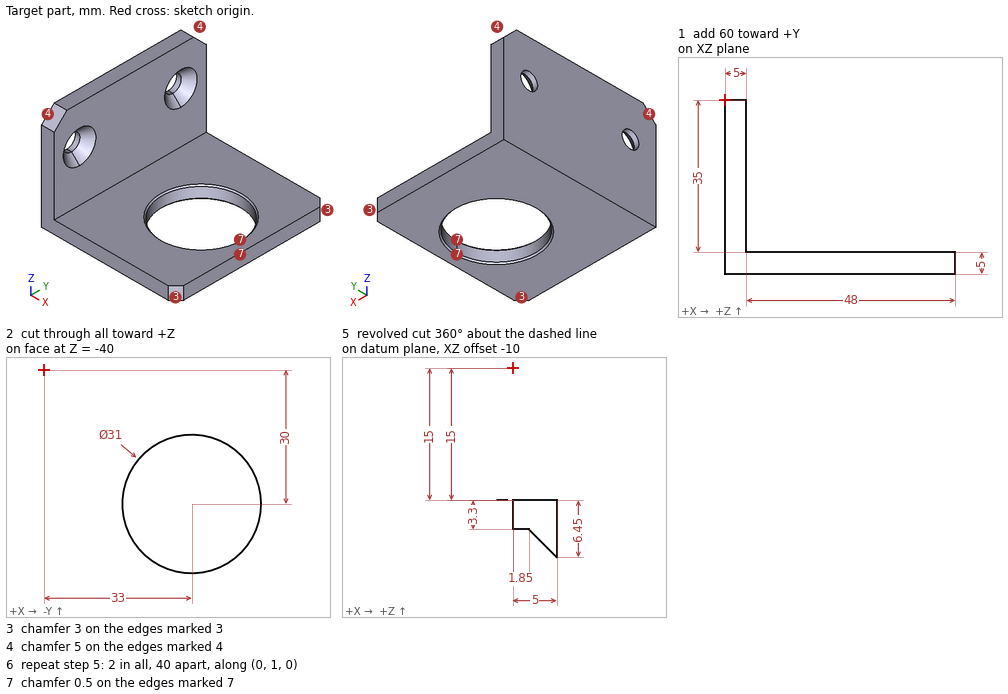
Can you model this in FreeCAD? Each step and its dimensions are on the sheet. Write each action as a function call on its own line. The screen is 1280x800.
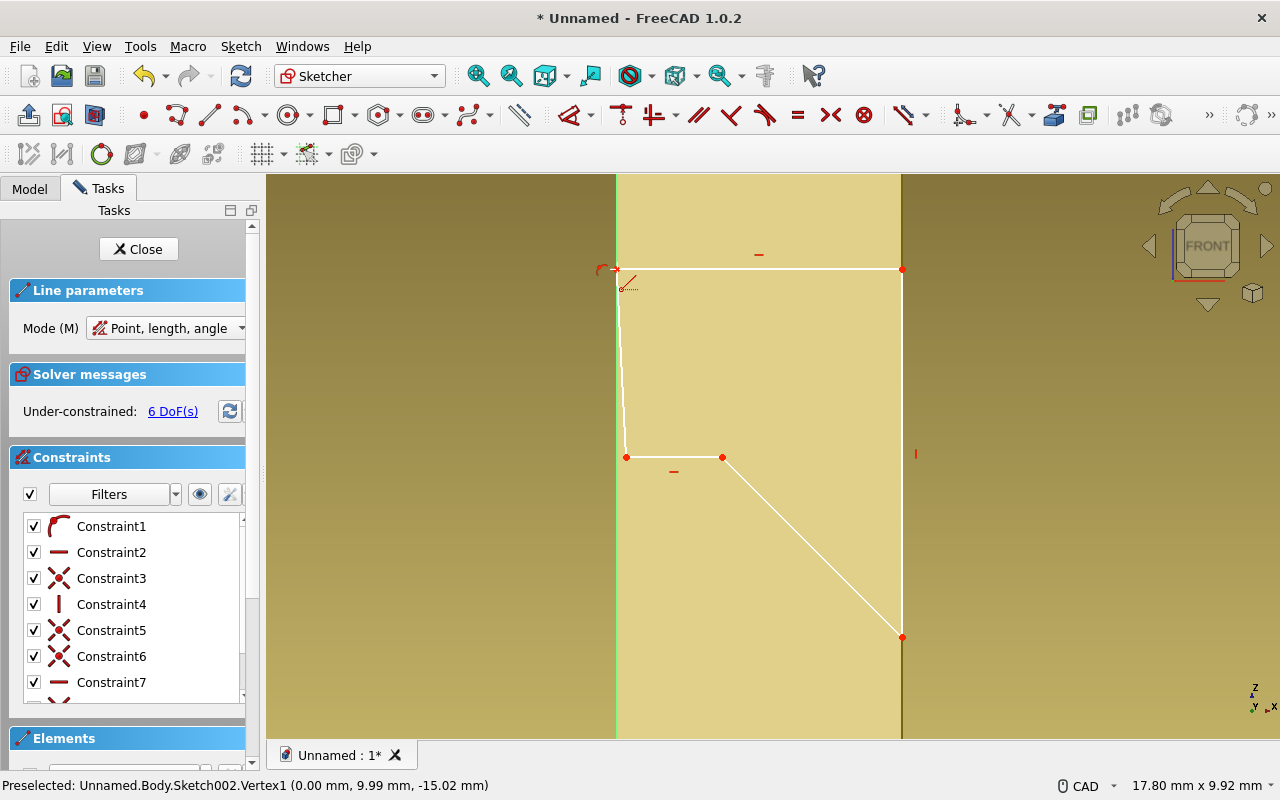
click(588, 268)
click(503, 268)
key(Escape)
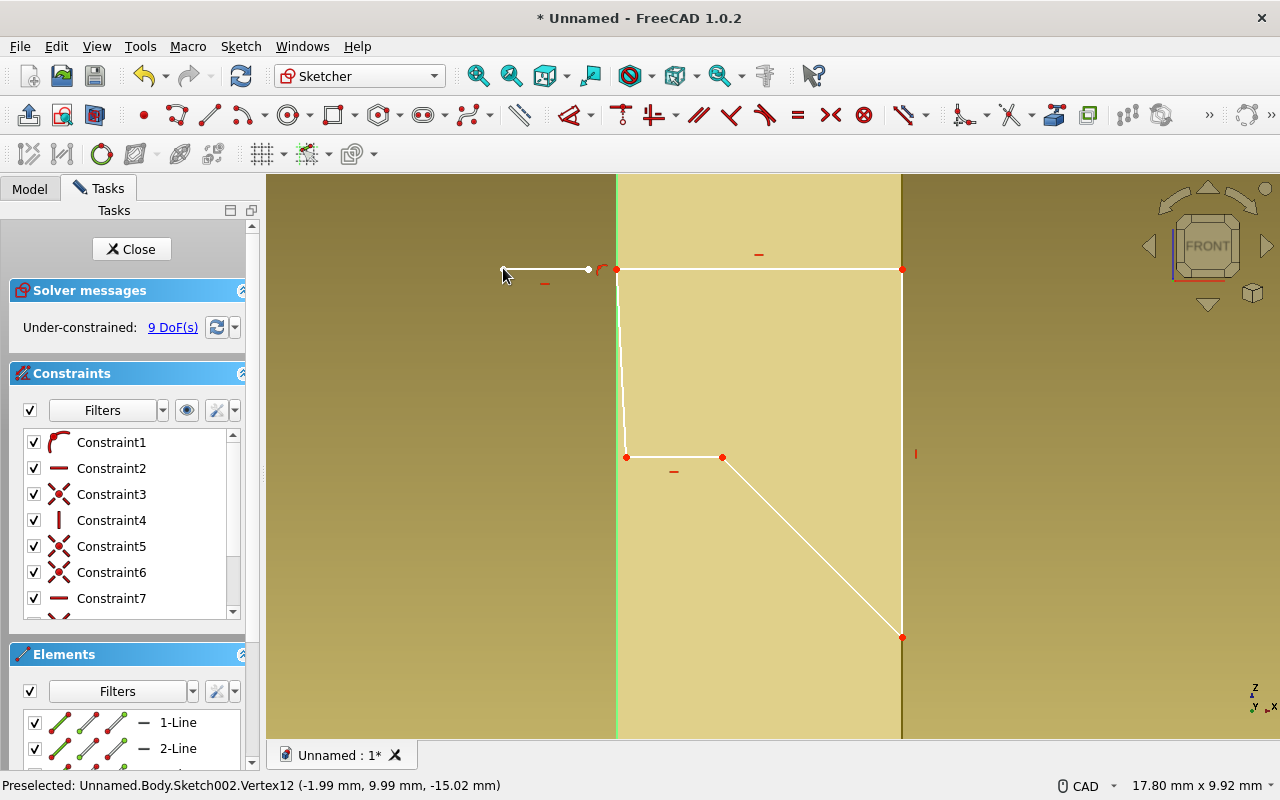
click(563, 269)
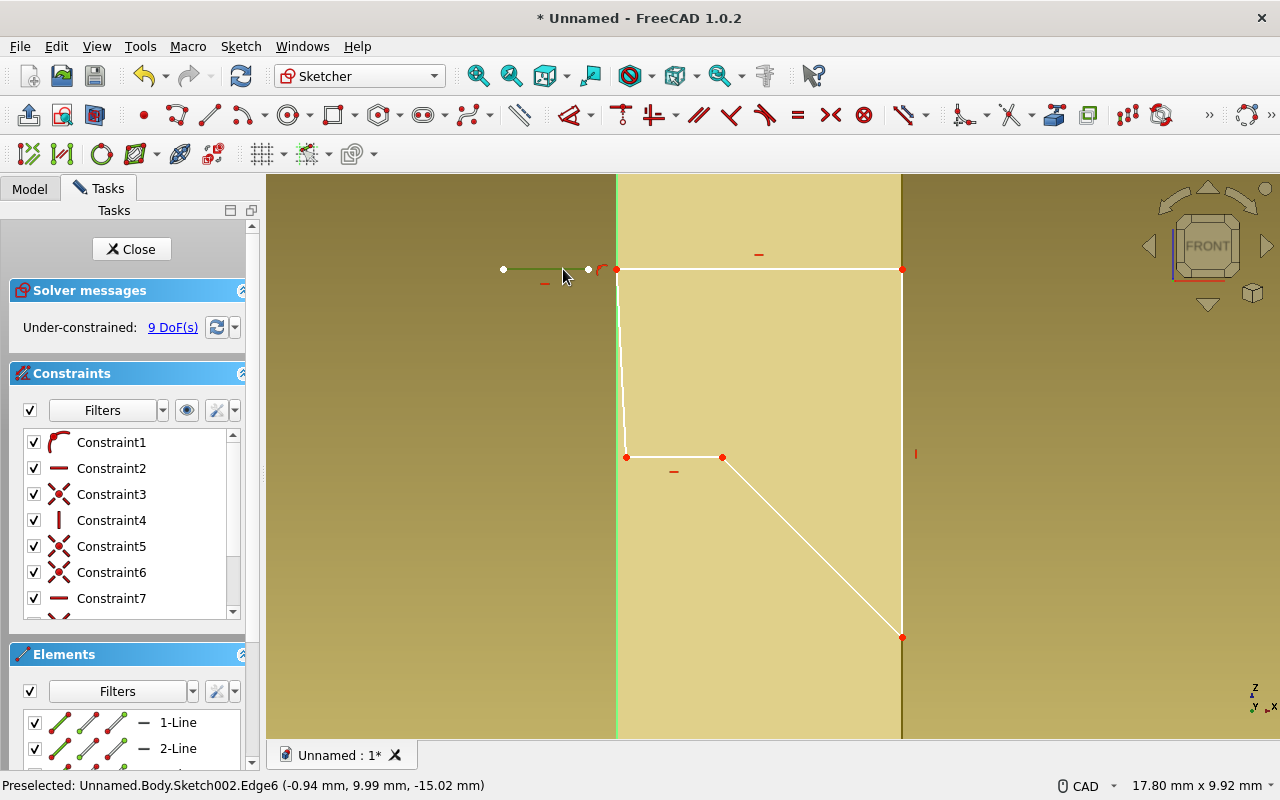
key(g)
key(n)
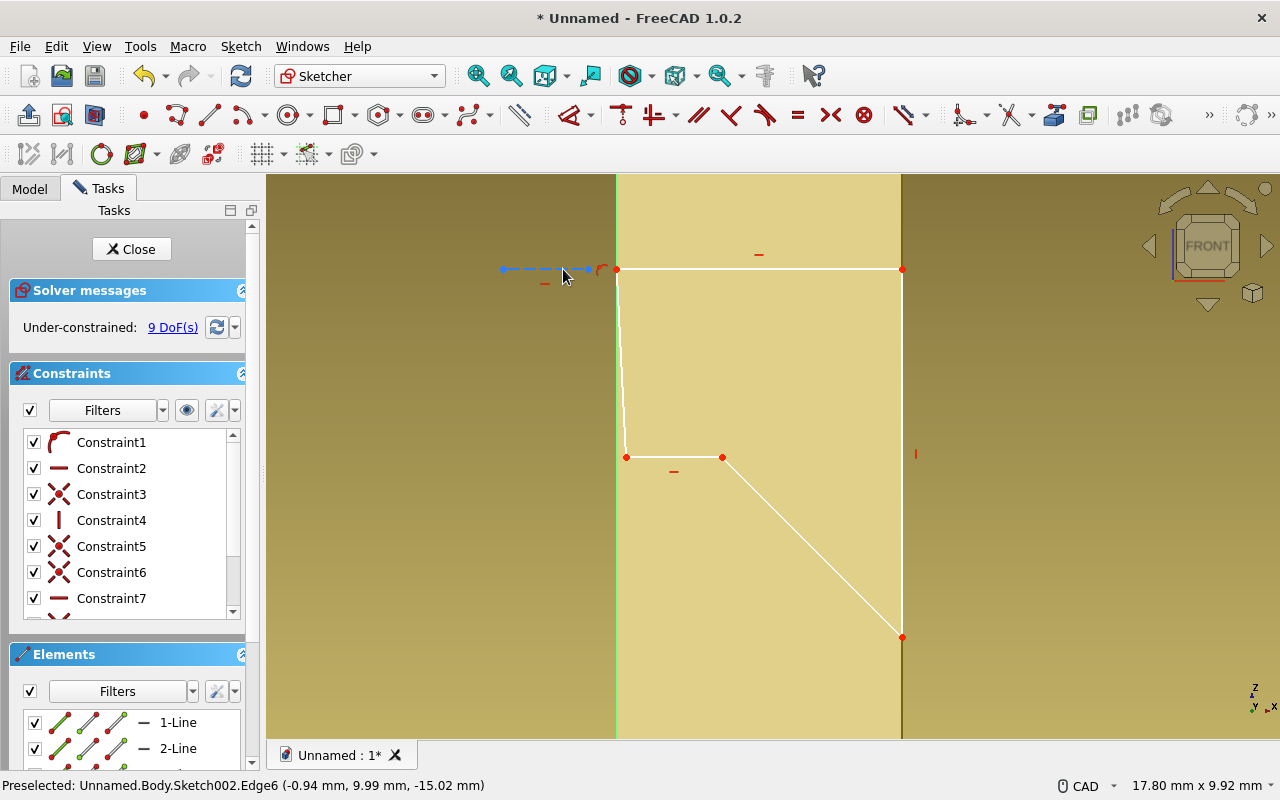
click(619, 325)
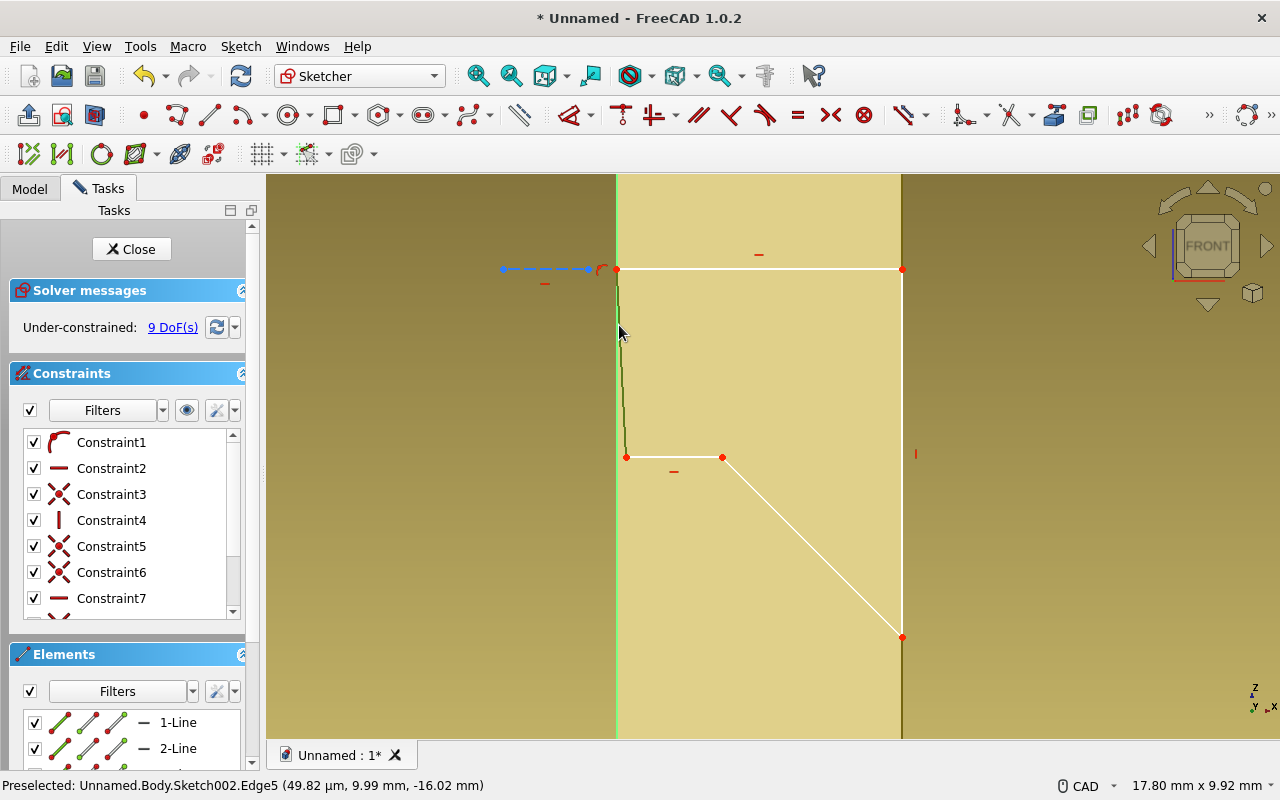
key(v)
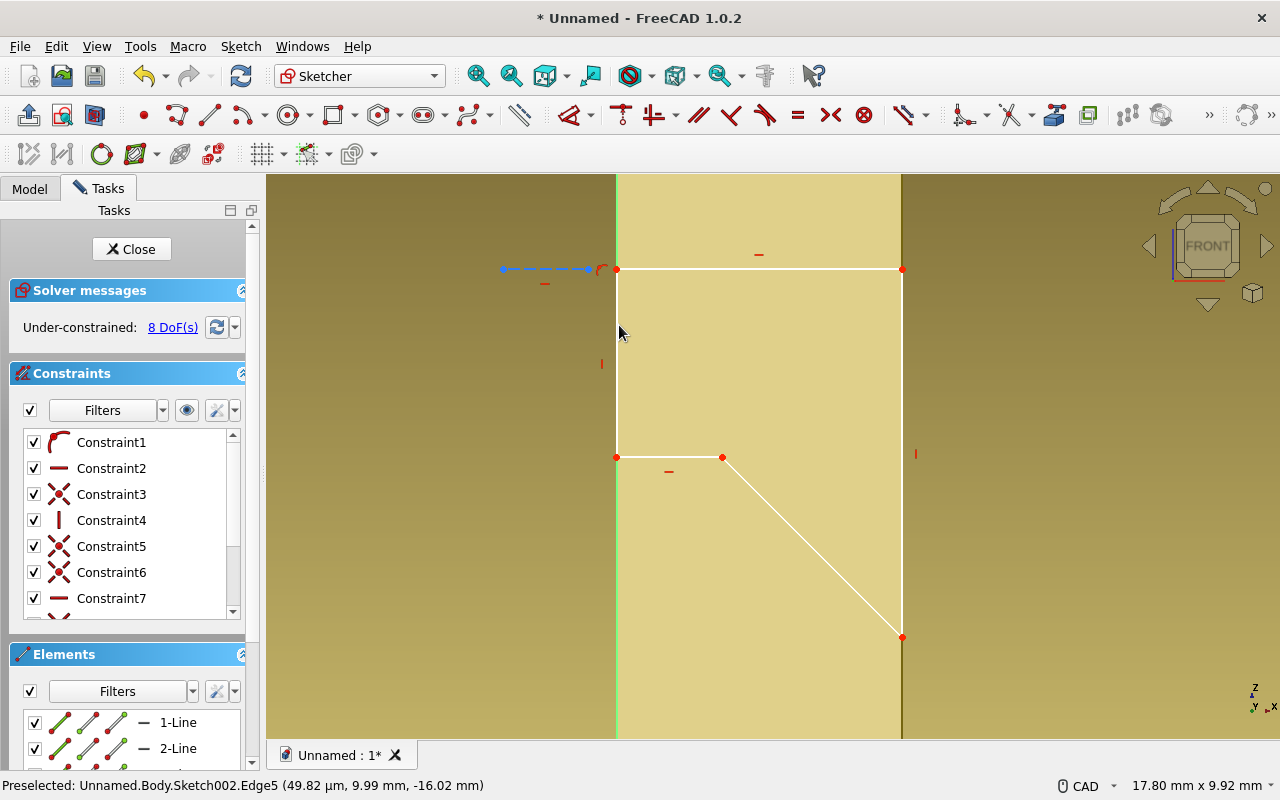
click(702, 269)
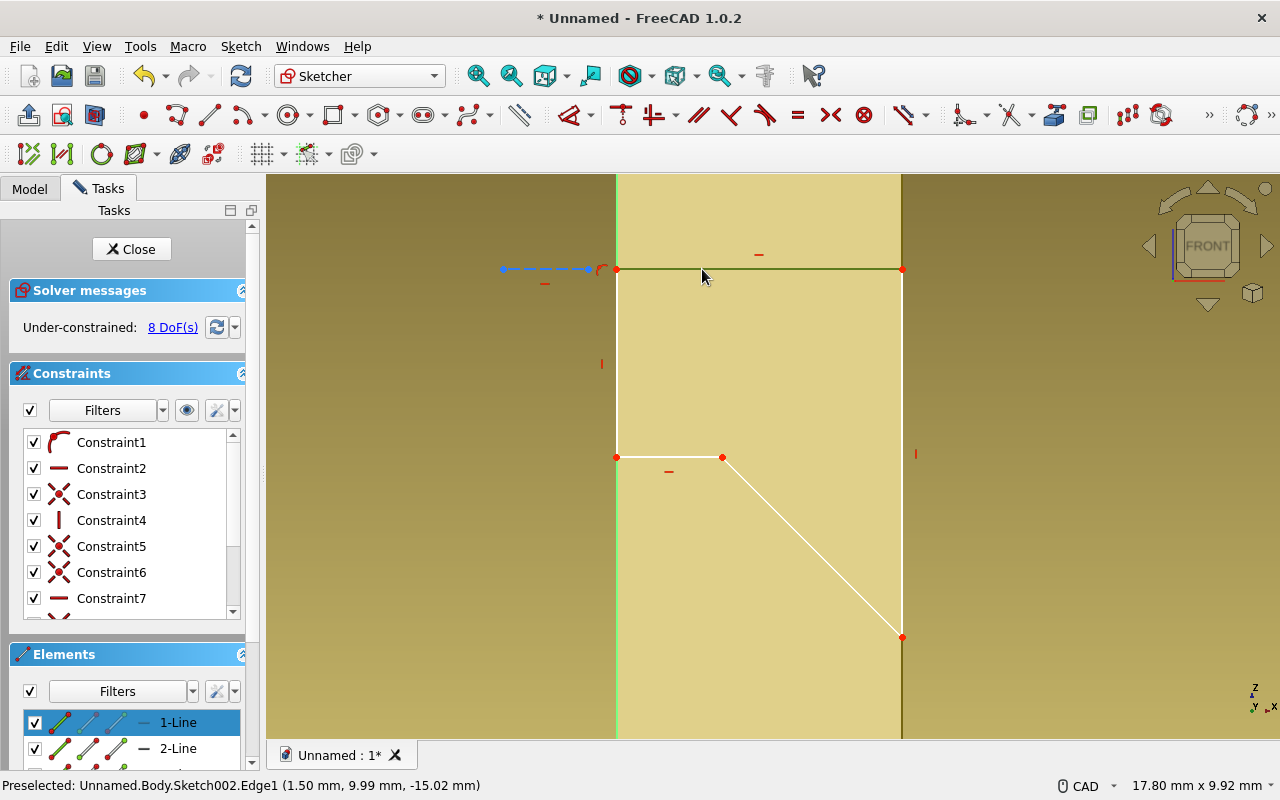
key(l)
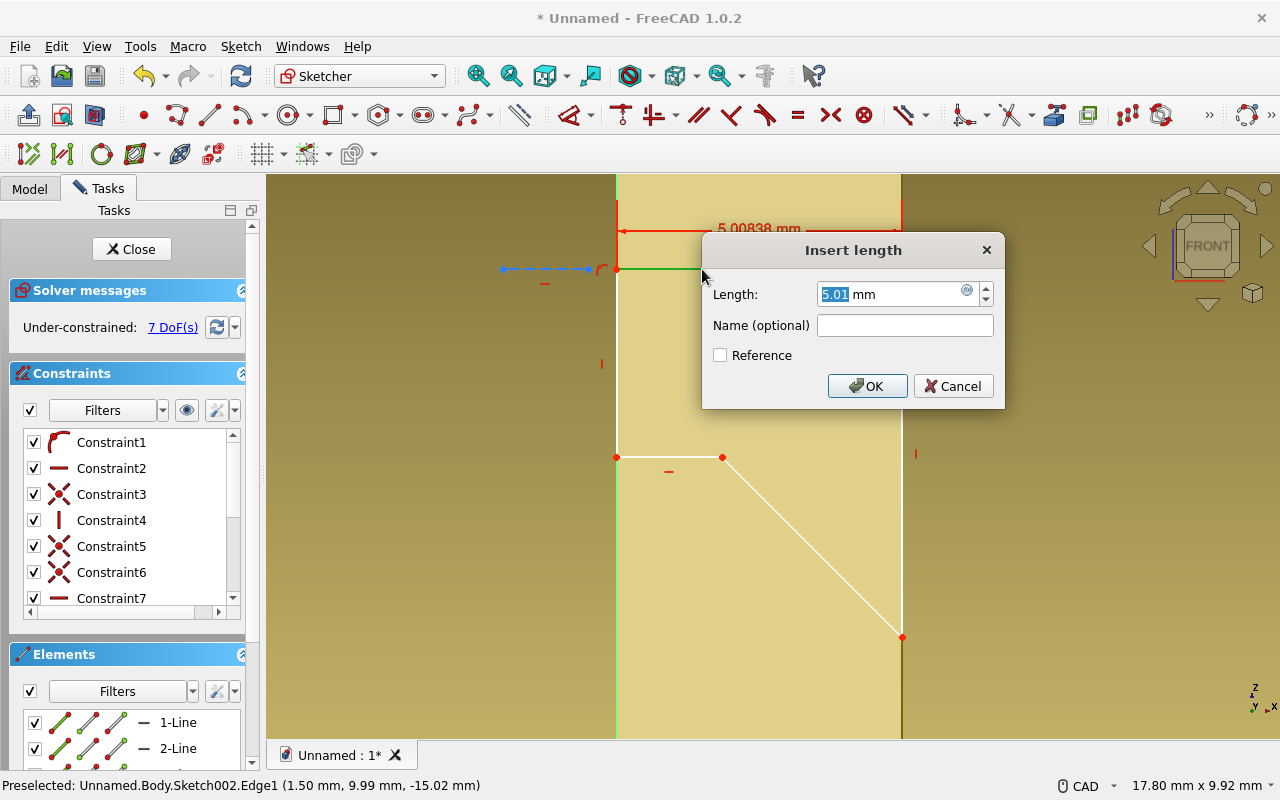
text(5)
key(Return)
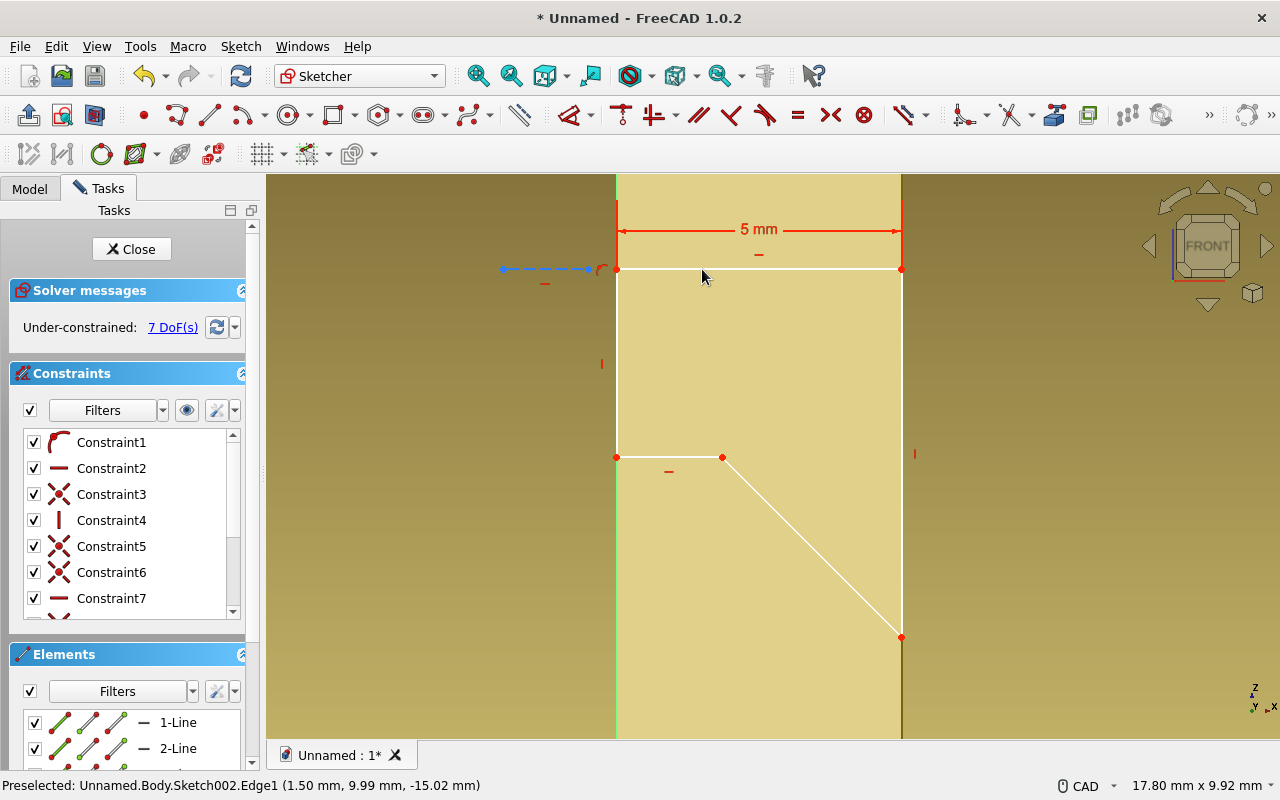
click(617, 401)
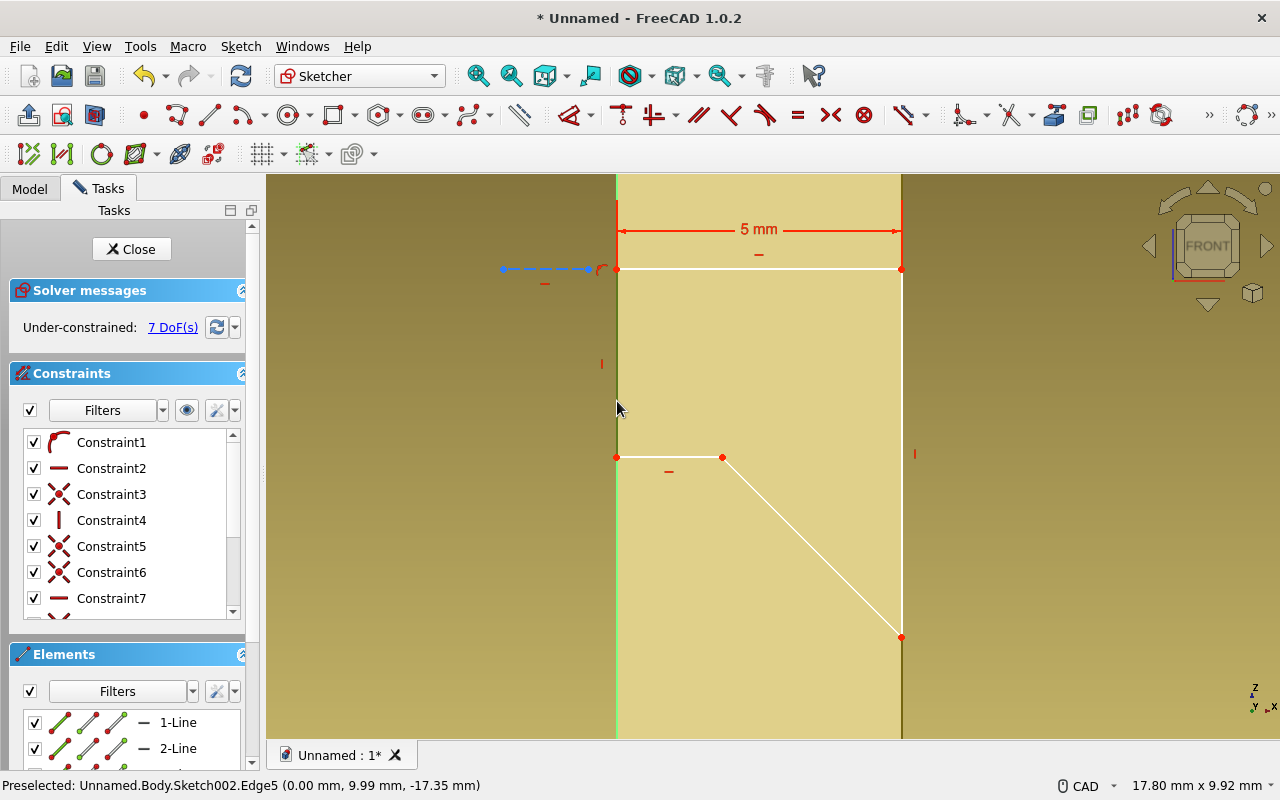
key(i)